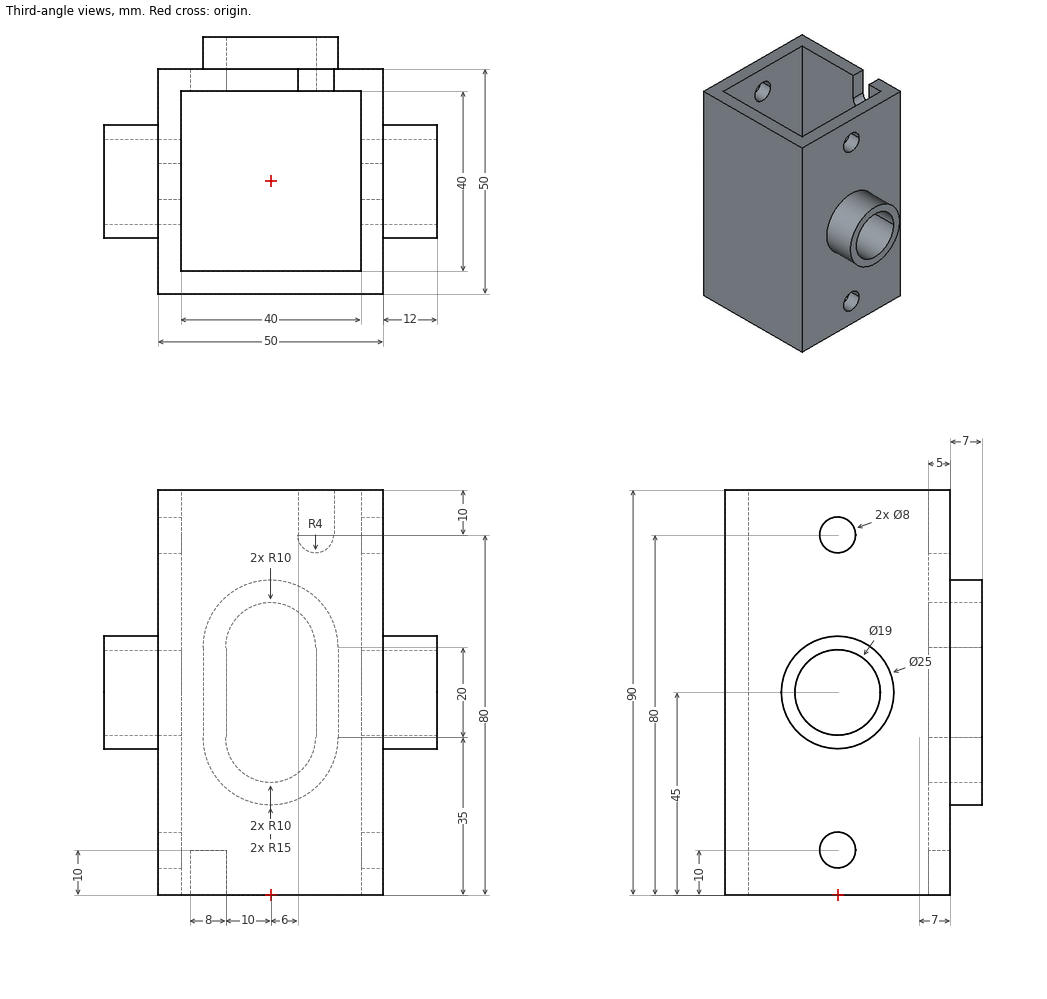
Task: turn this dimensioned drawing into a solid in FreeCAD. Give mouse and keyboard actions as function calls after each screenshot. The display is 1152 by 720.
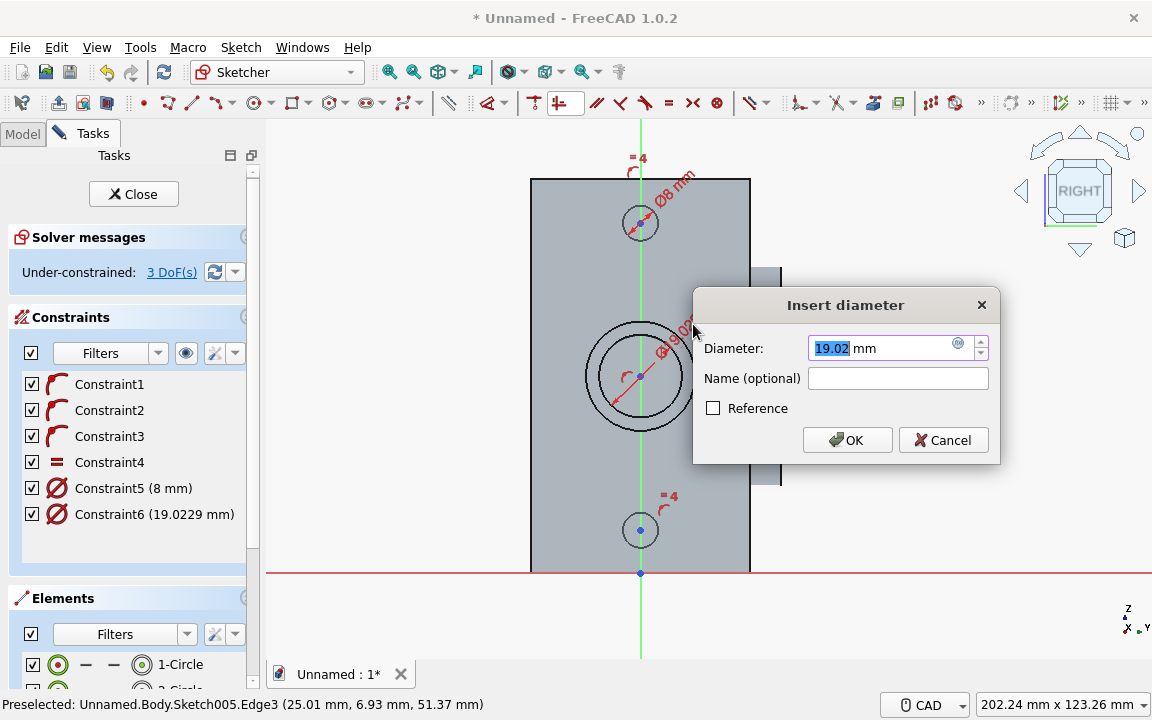
text(19)
key(Return)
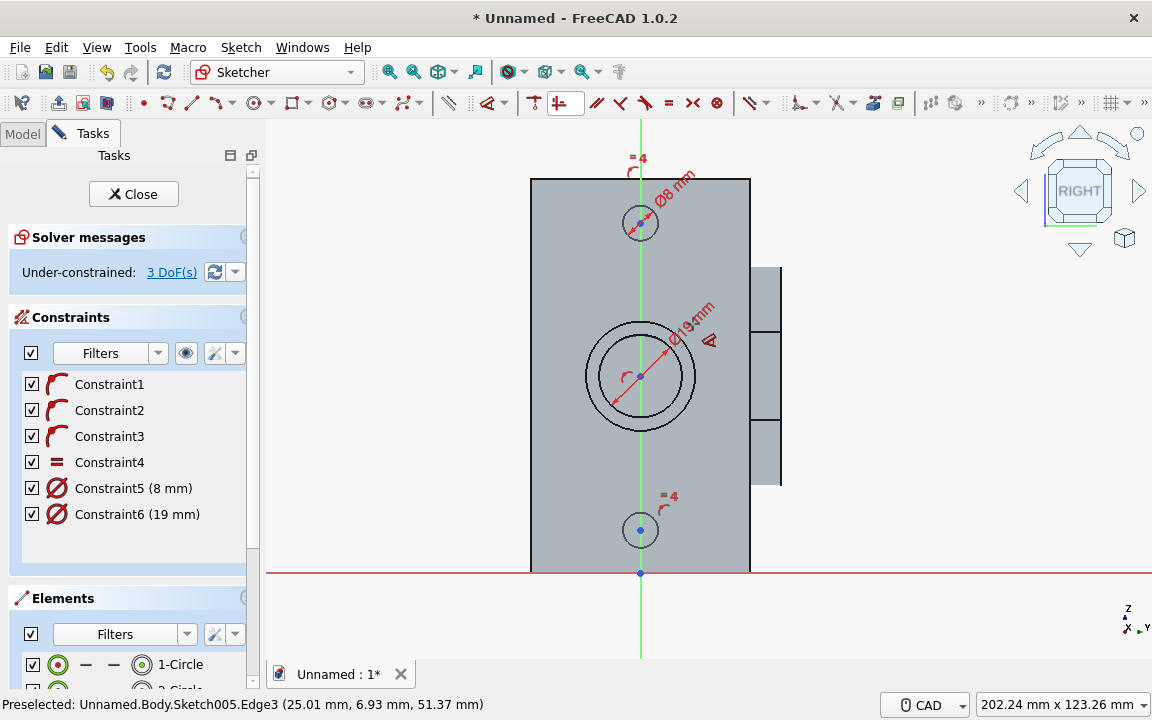
click(641, 223)
click(675, 479)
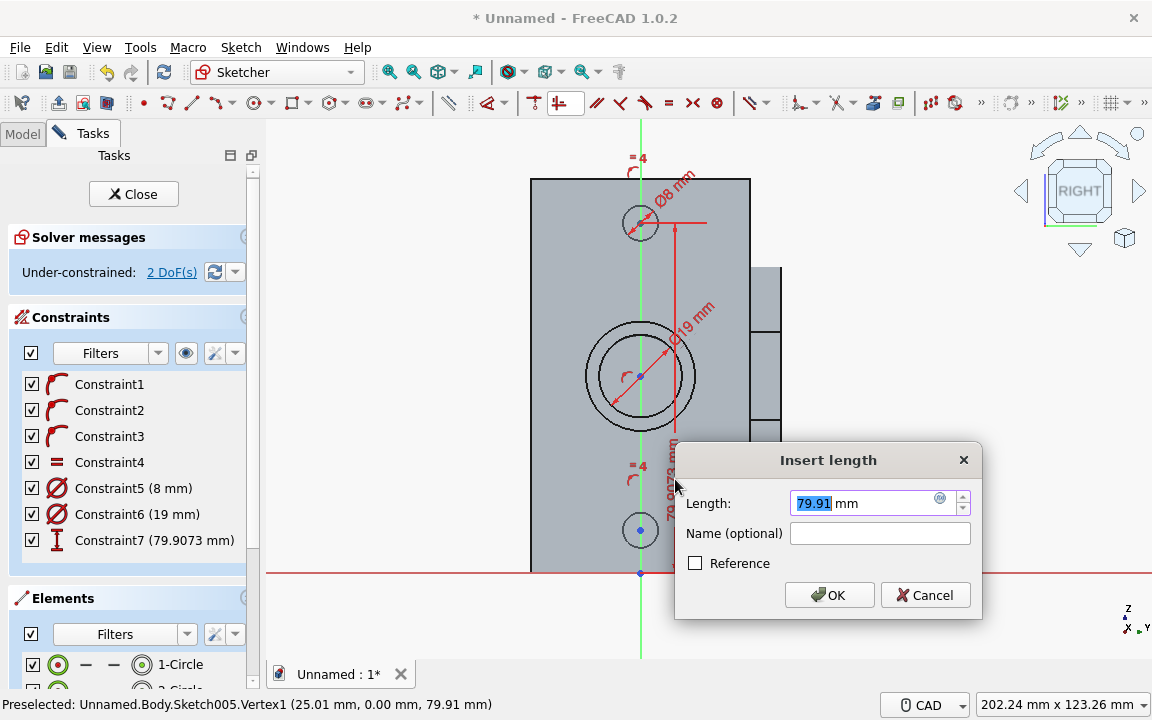
text(80)
key(Return)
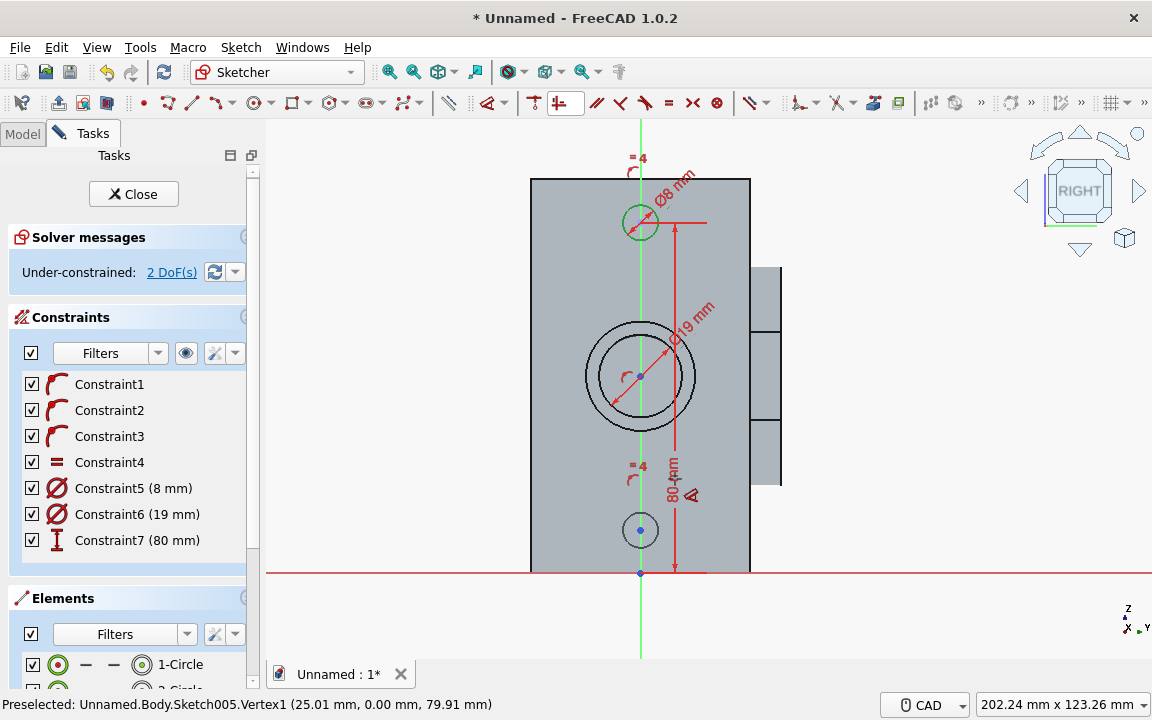
click(641, 530)
click(675, 552)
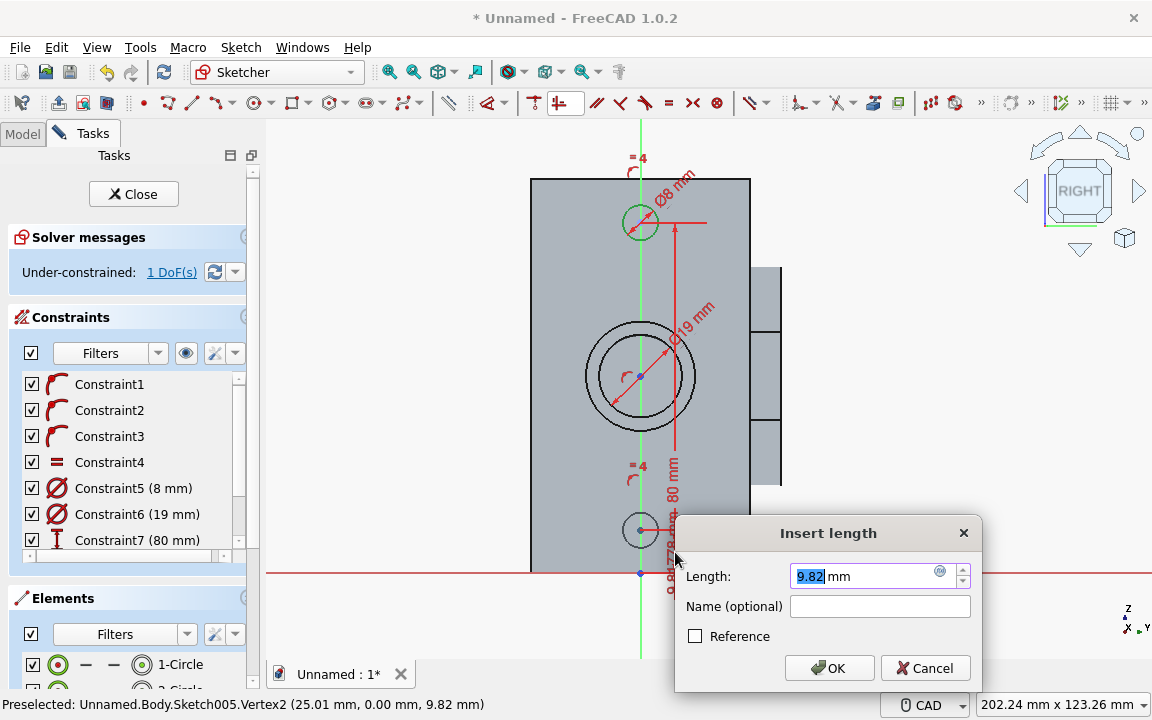
text(10)
key(Return)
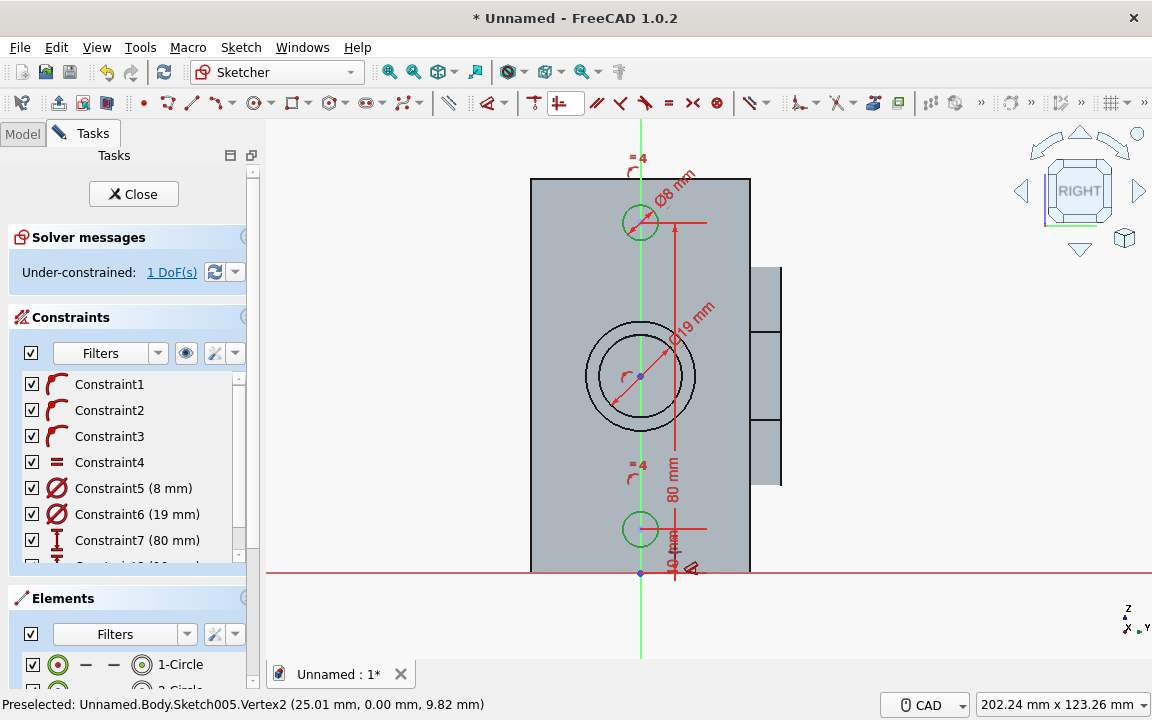
click(641, 377)
click(675, 430)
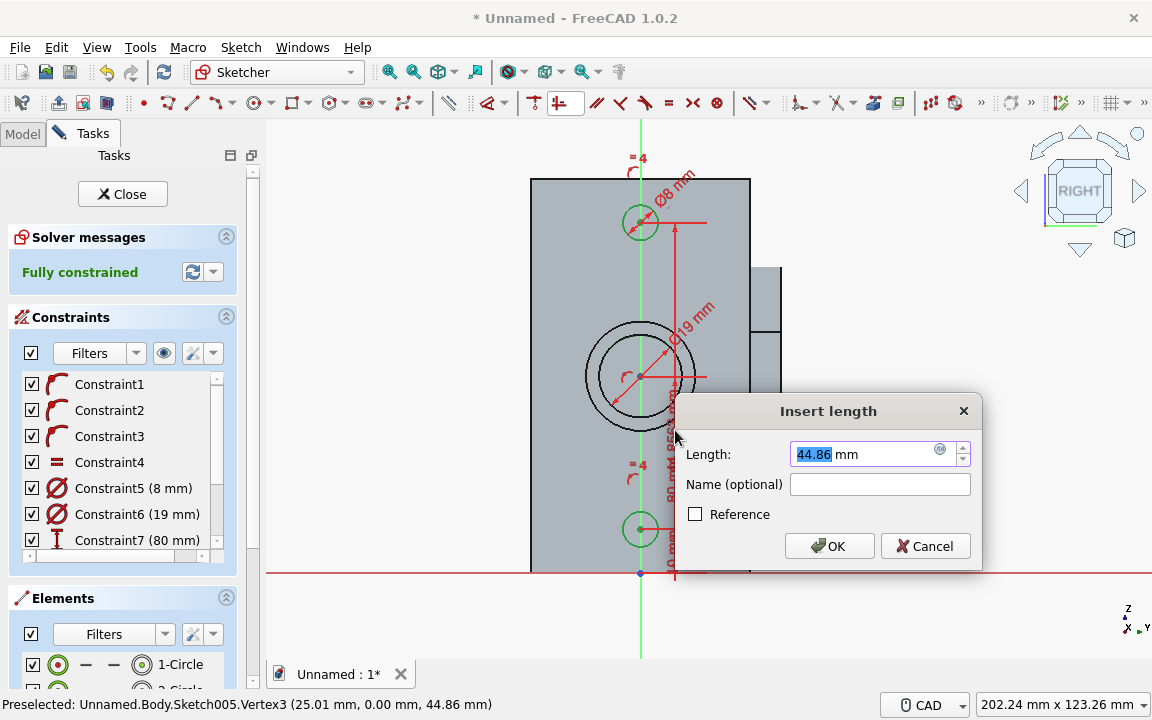
text(45)
key(Return)
key(Escape)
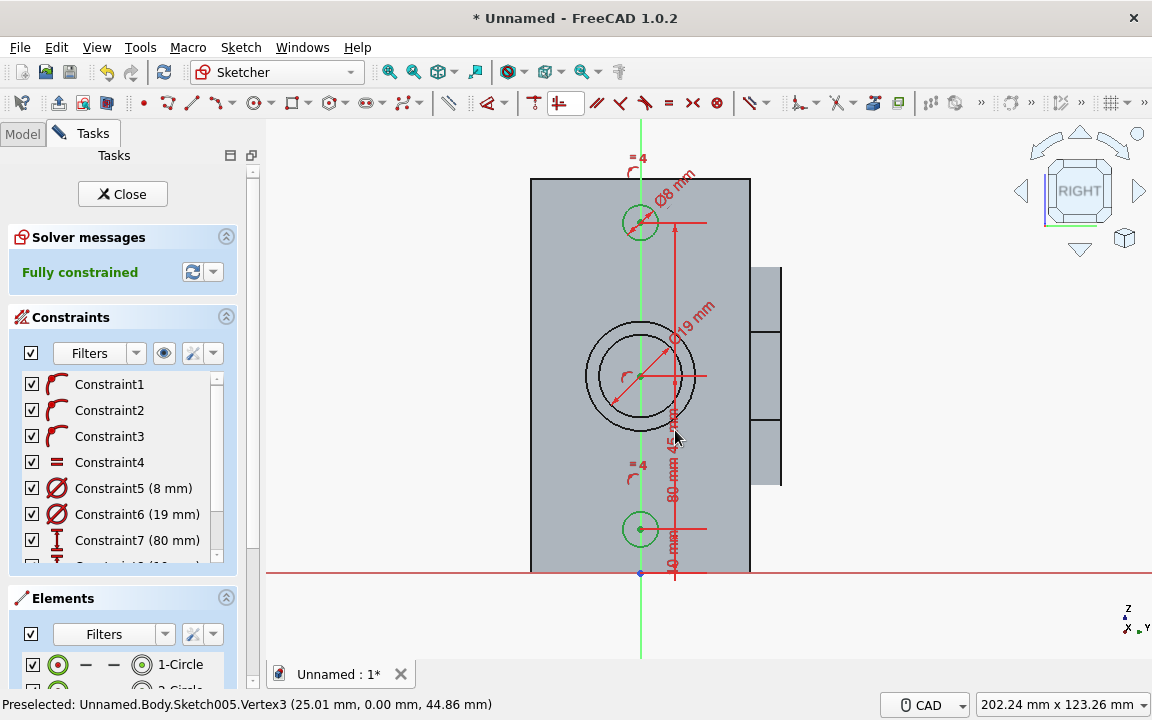
click(123, 194)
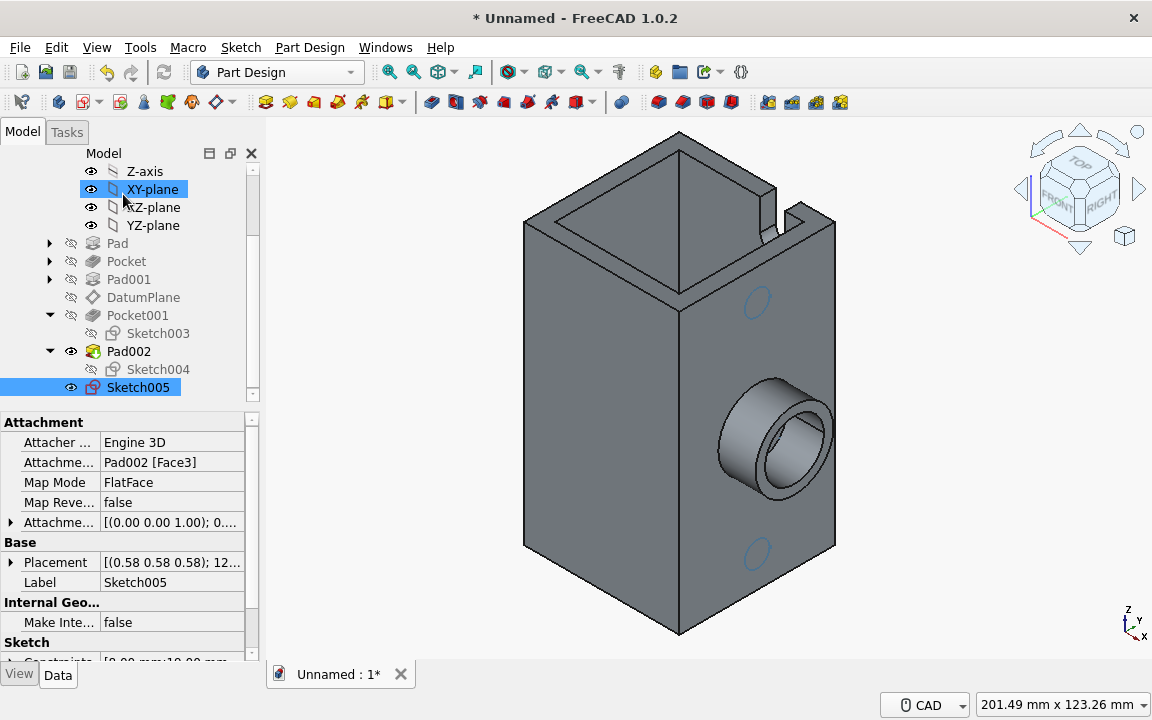
click(432, 102)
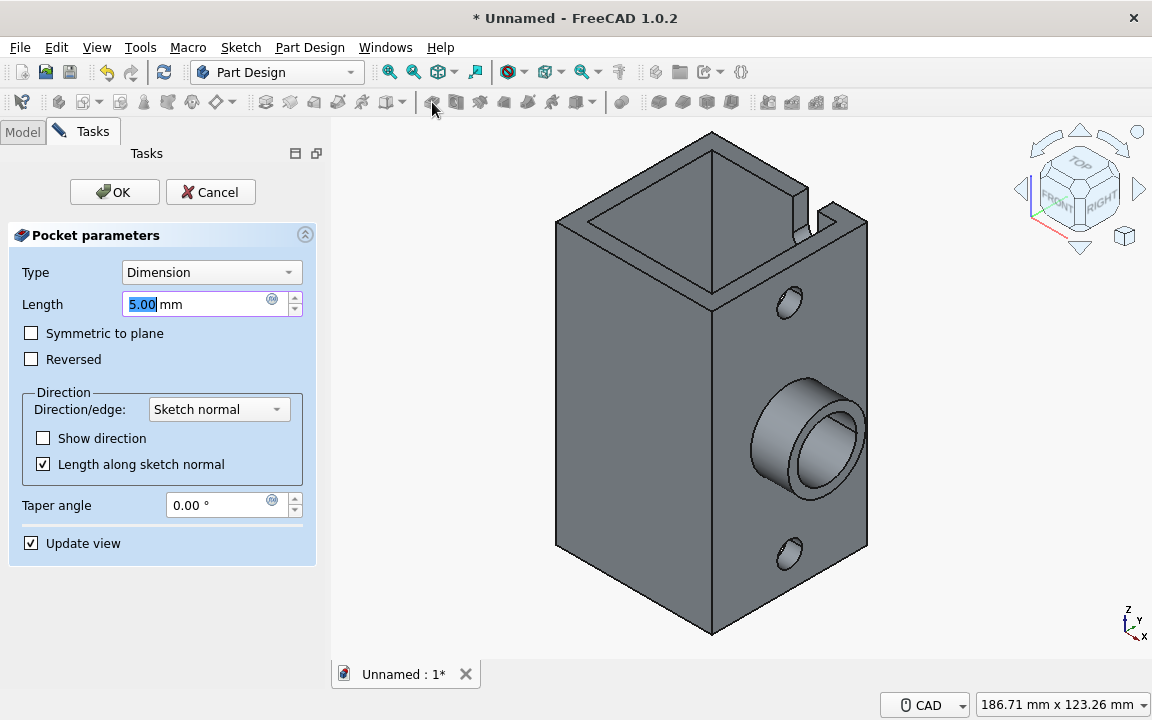
click(212, 272)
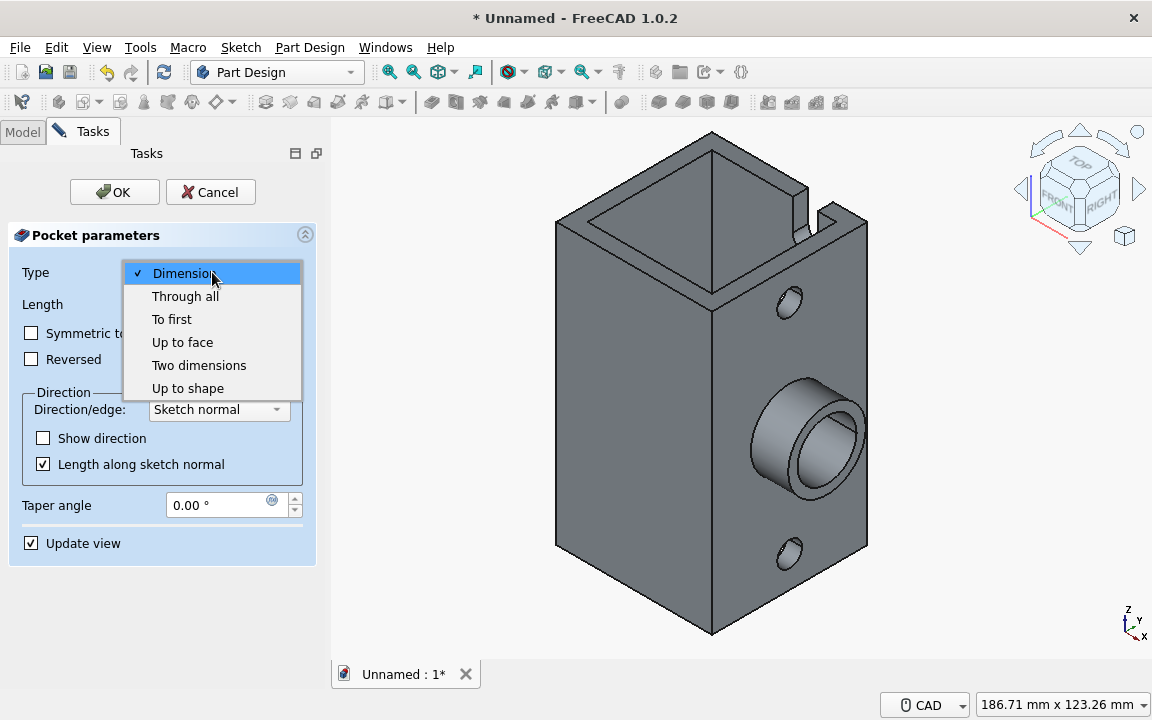
click(212, 296)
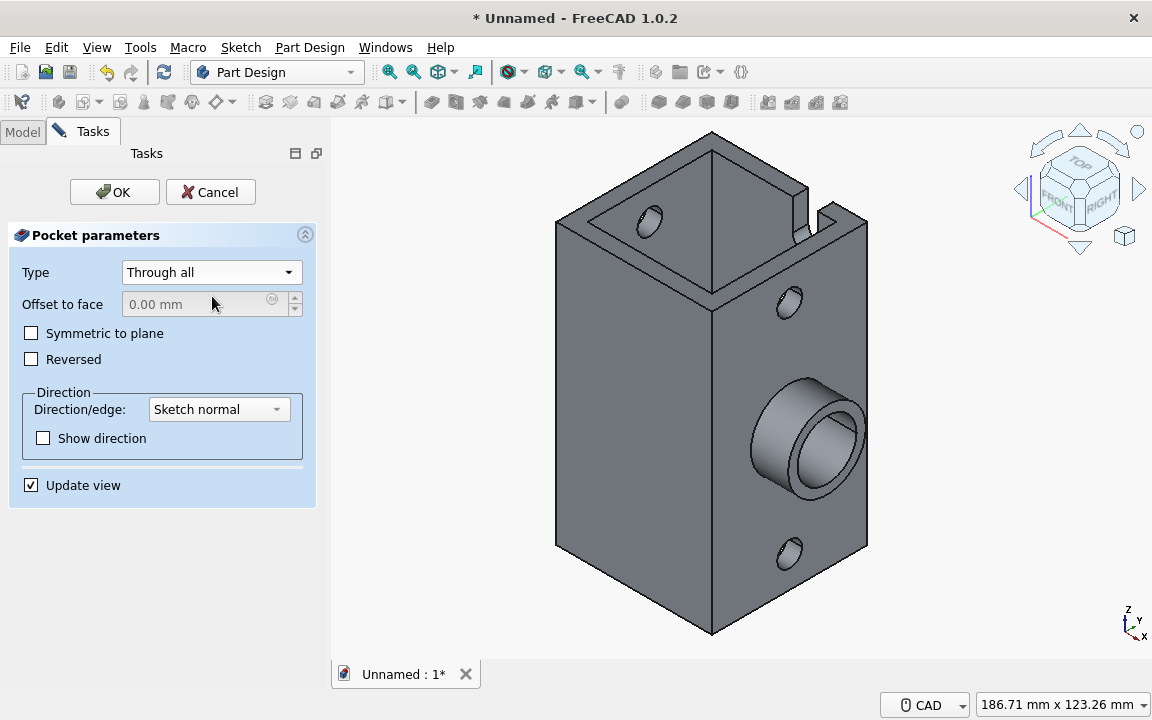
click(115, 192)